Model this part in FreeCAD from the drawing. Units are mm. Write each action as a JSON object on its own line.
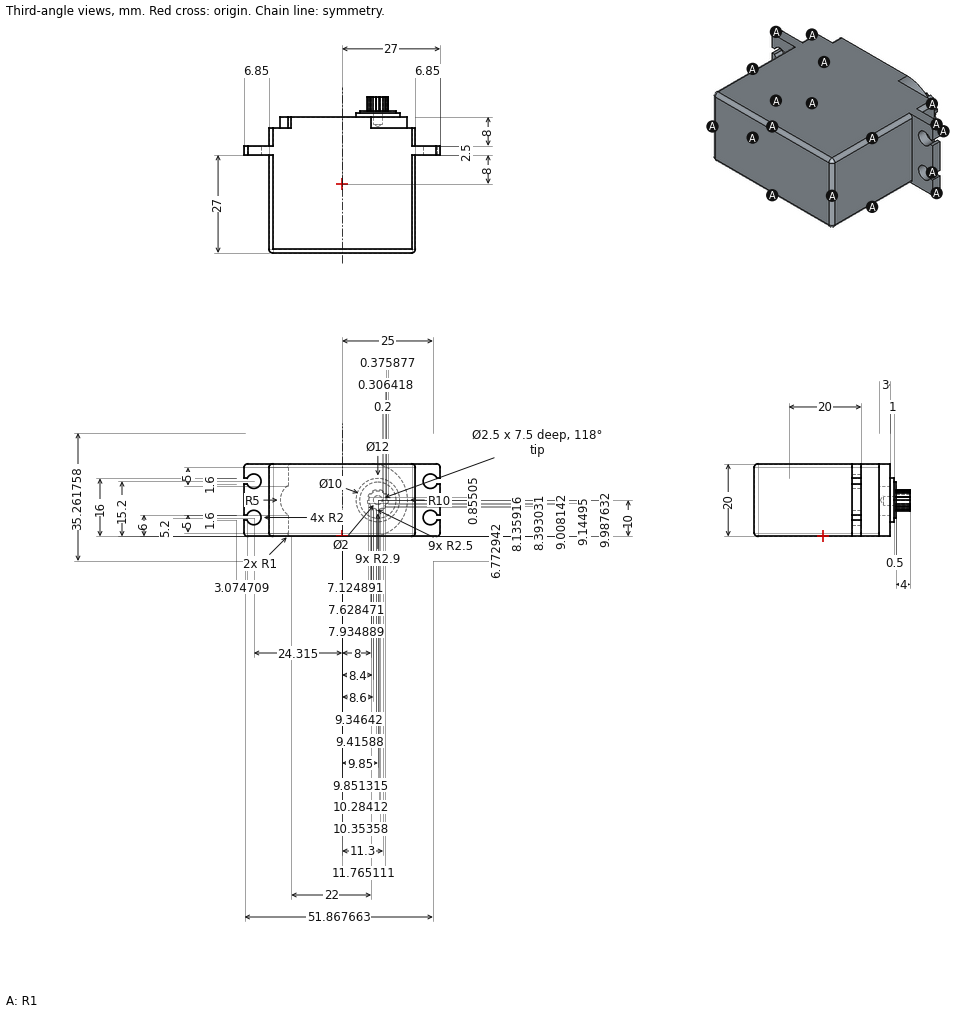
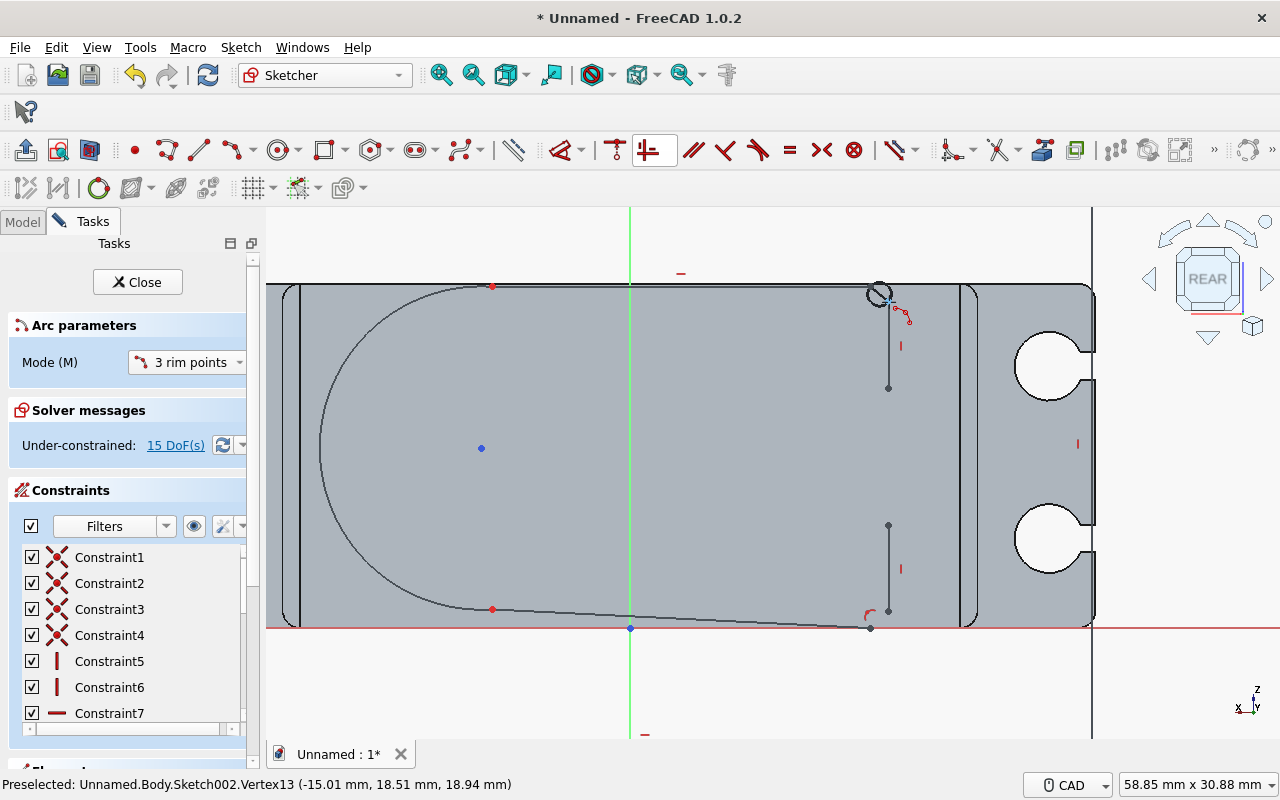
{"action": "scroll", "coordinate": [883, 289], "scroll_direction": "up", "scroll_amount": 6}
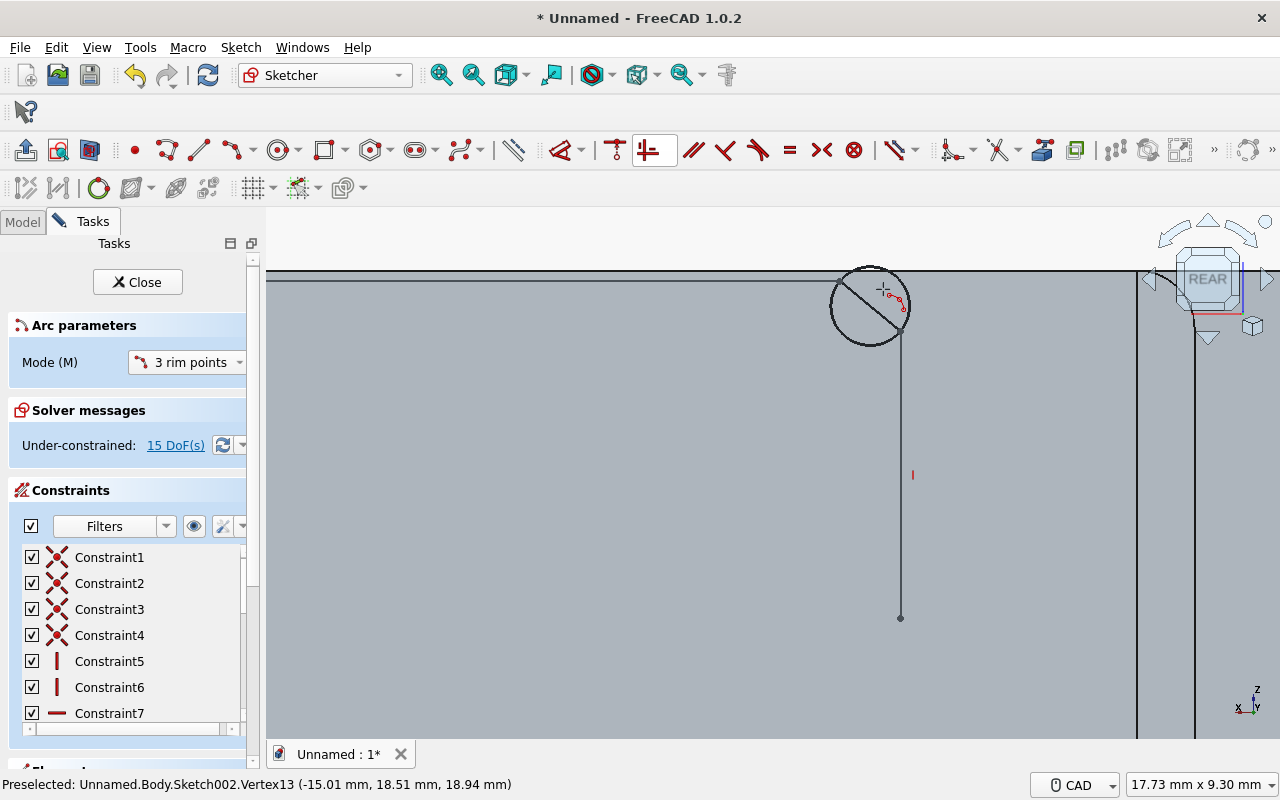
{"action": "left_click", "coordinate": [883, 287]}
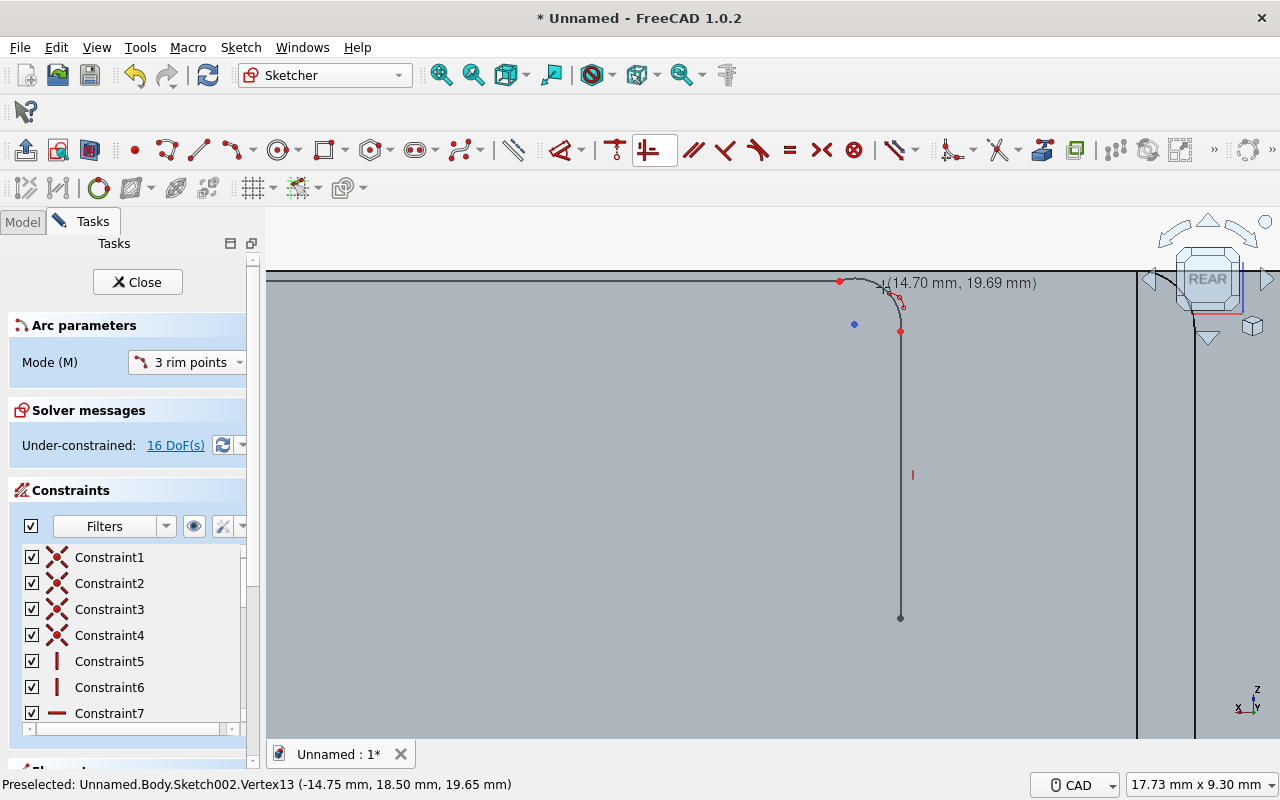
{"action": "scroll", "coordinate": [825, 410], "scroll_direction": "down", "scroll_amount": 9}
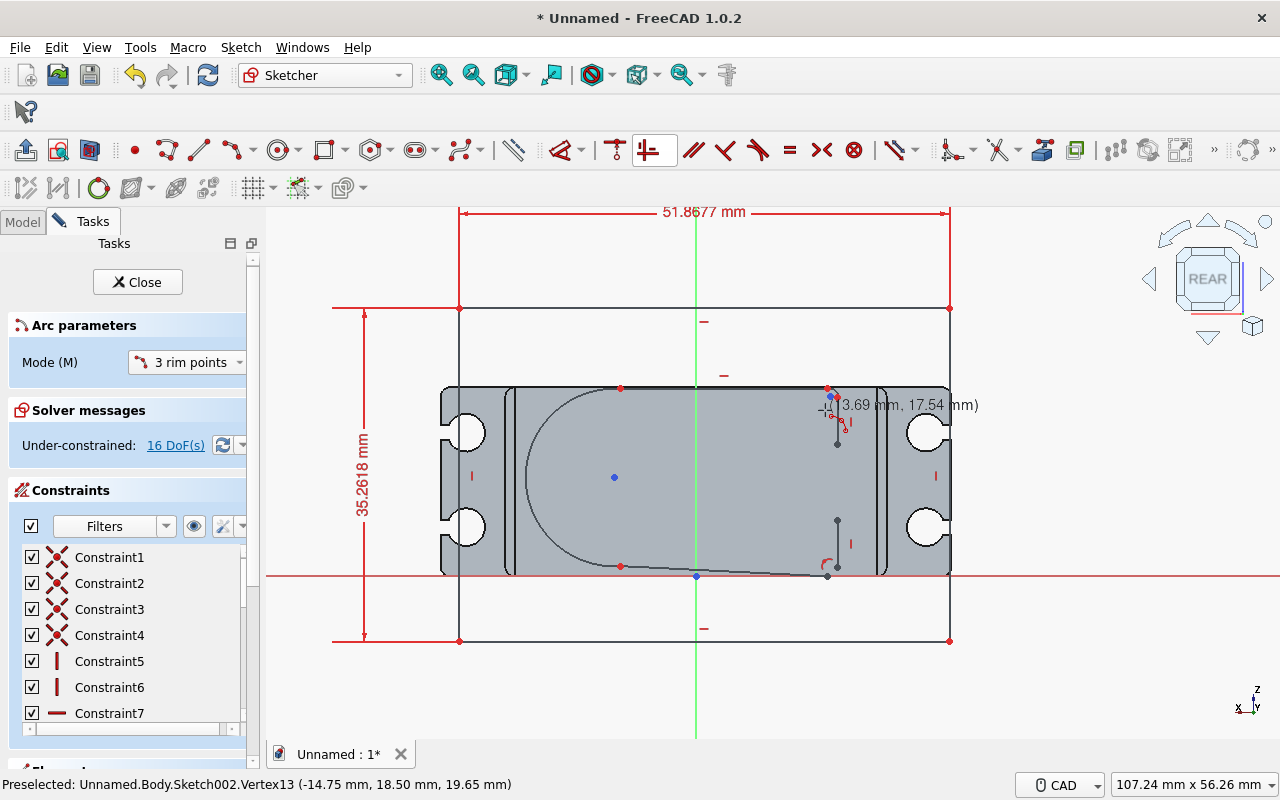
{"action": "left_click", "coordinate": [838, 445]}
{"action": "left_click", "coordinate": [838, 520]}
{"action": "left_click", "coordinate": [857, 482]}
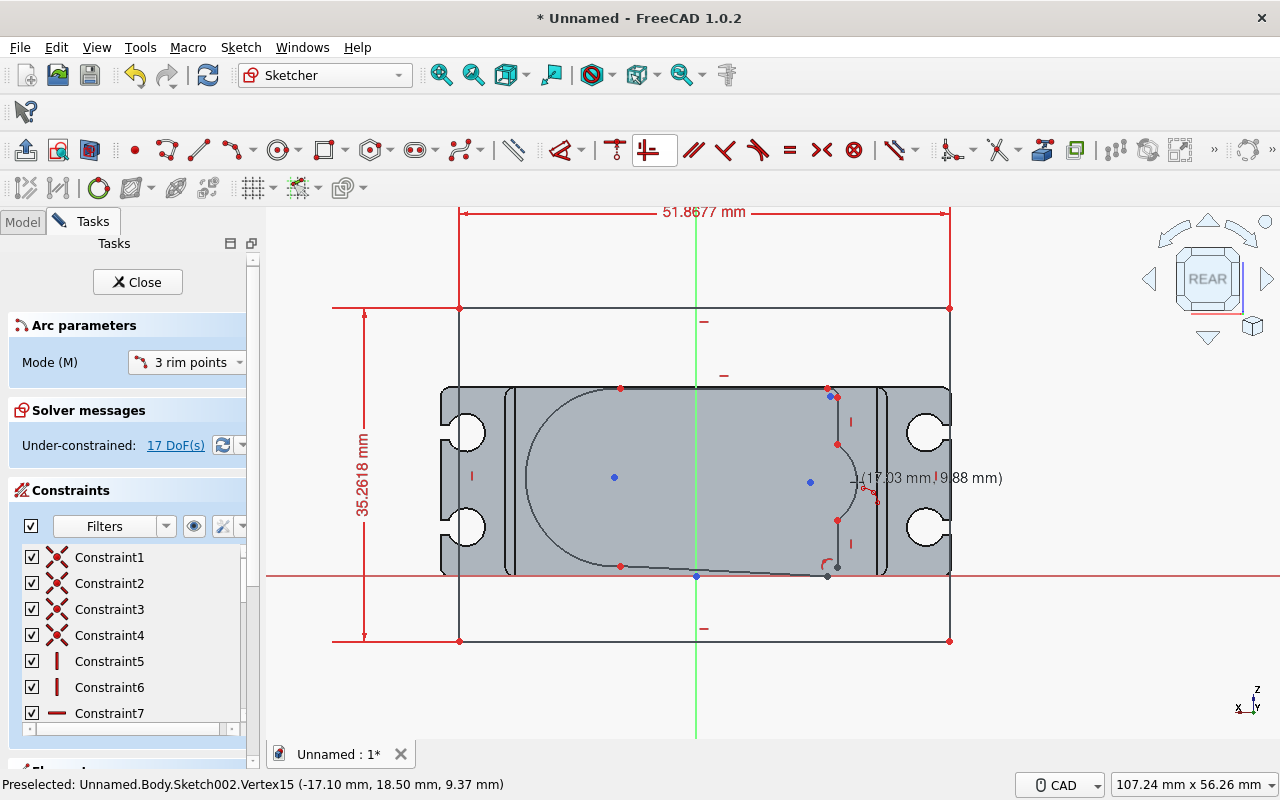
{"action": "scroll", "coordinate": [838, 567], "scroll_direction": "up", "scroll_amount": 3}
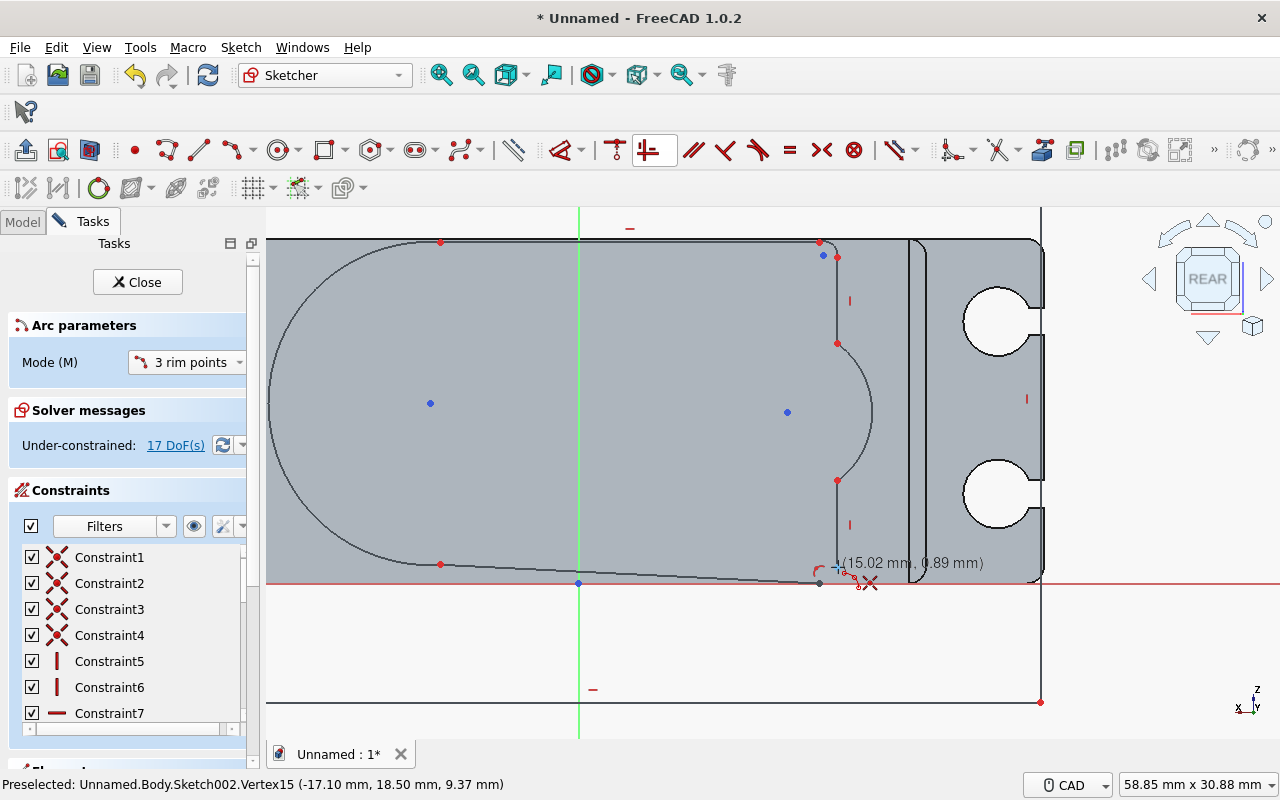
{"action": "left_click", "coordinate": [837, 567]}
{"action": "left_click", "coordinate": [819, 584]}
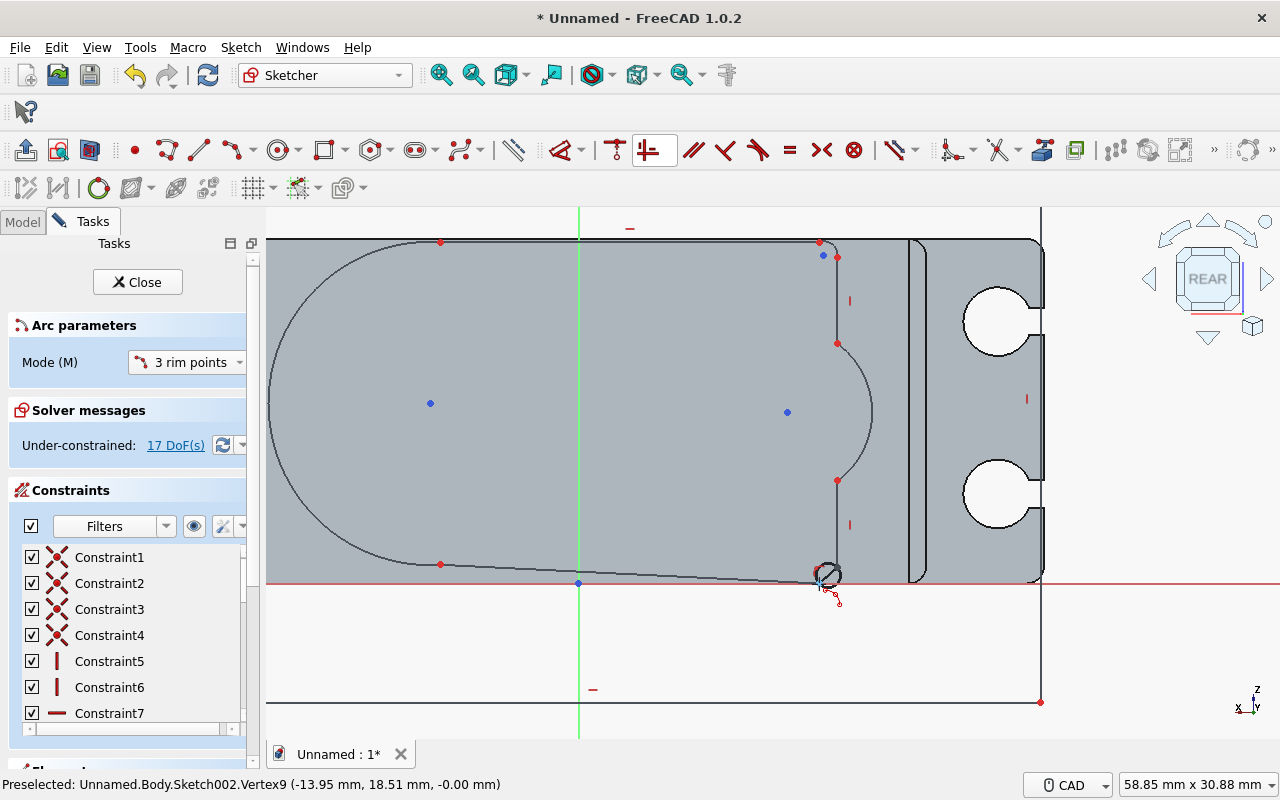
{"action": "scroll", "coordinate": [832, 578], "scroll_direction": "up", "scroll_amount": 6}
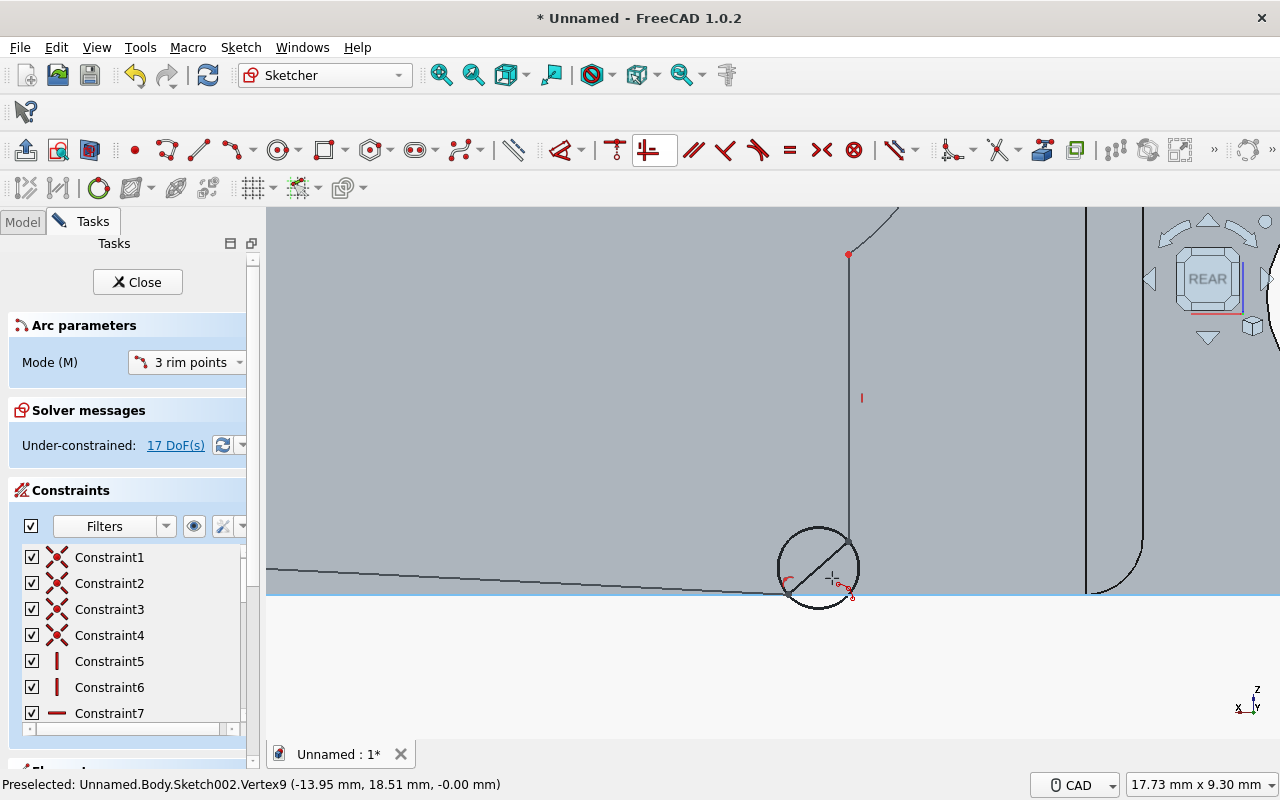
{"action": "left_click", "coordinate": [831, 578]}
{"action": "key", "text": "Escape"}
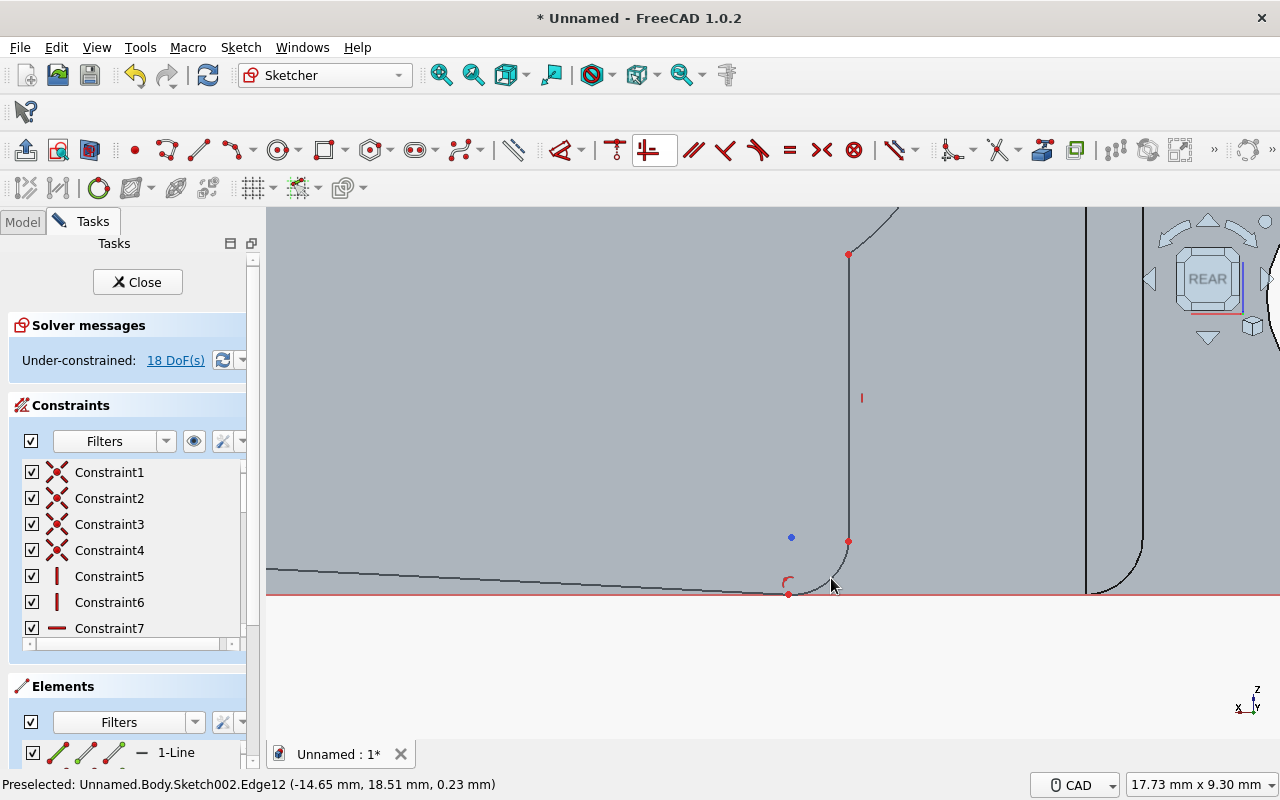
{"action": "left_click", "coordinate": [411, 576]}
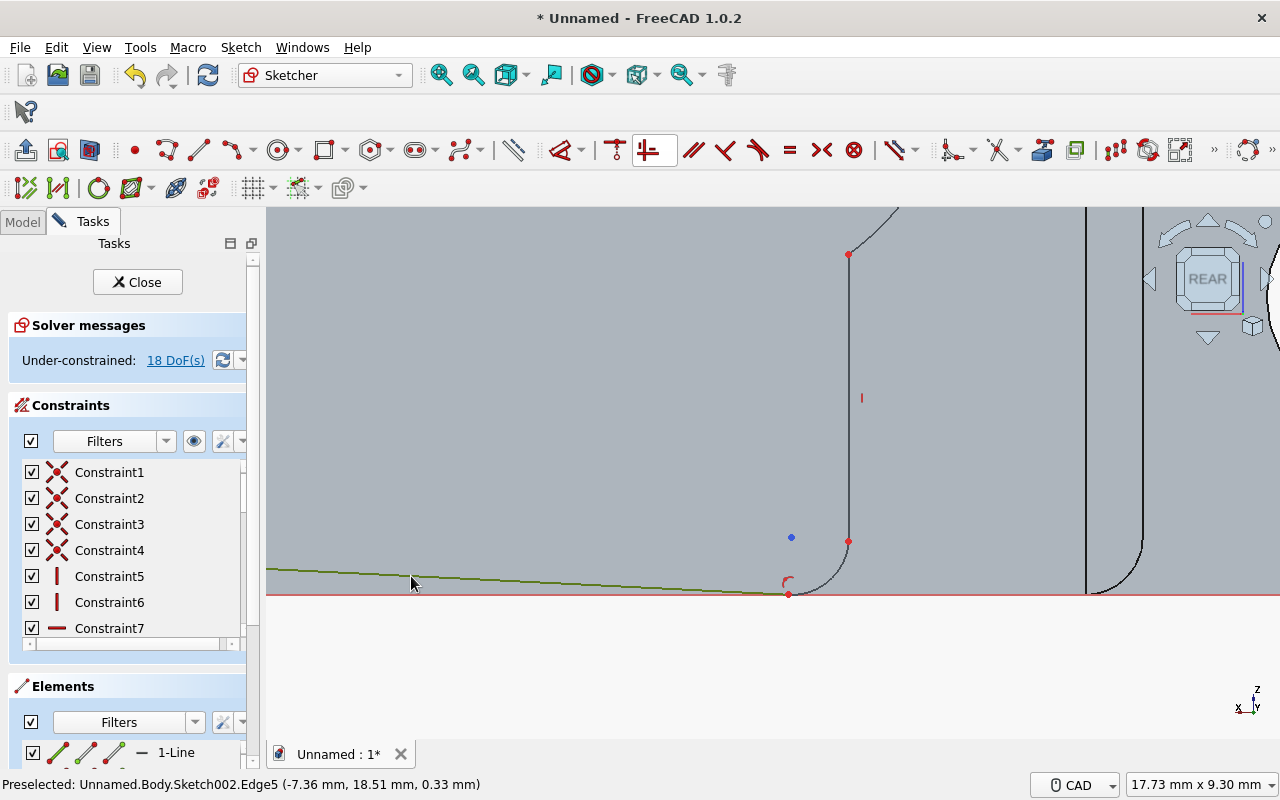
{"action": "scroll", "coordinate": [835, 572], "scroll_direction": "down", "scroll_amount": 9}